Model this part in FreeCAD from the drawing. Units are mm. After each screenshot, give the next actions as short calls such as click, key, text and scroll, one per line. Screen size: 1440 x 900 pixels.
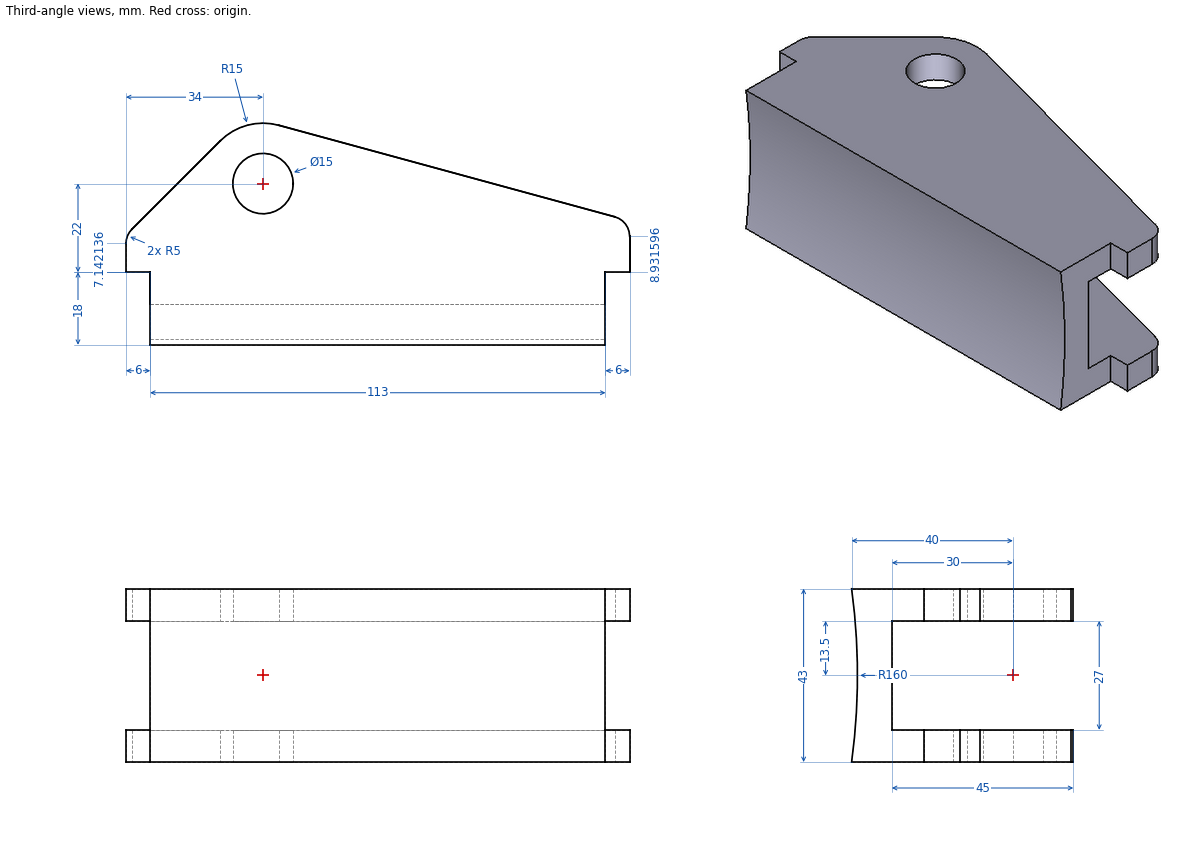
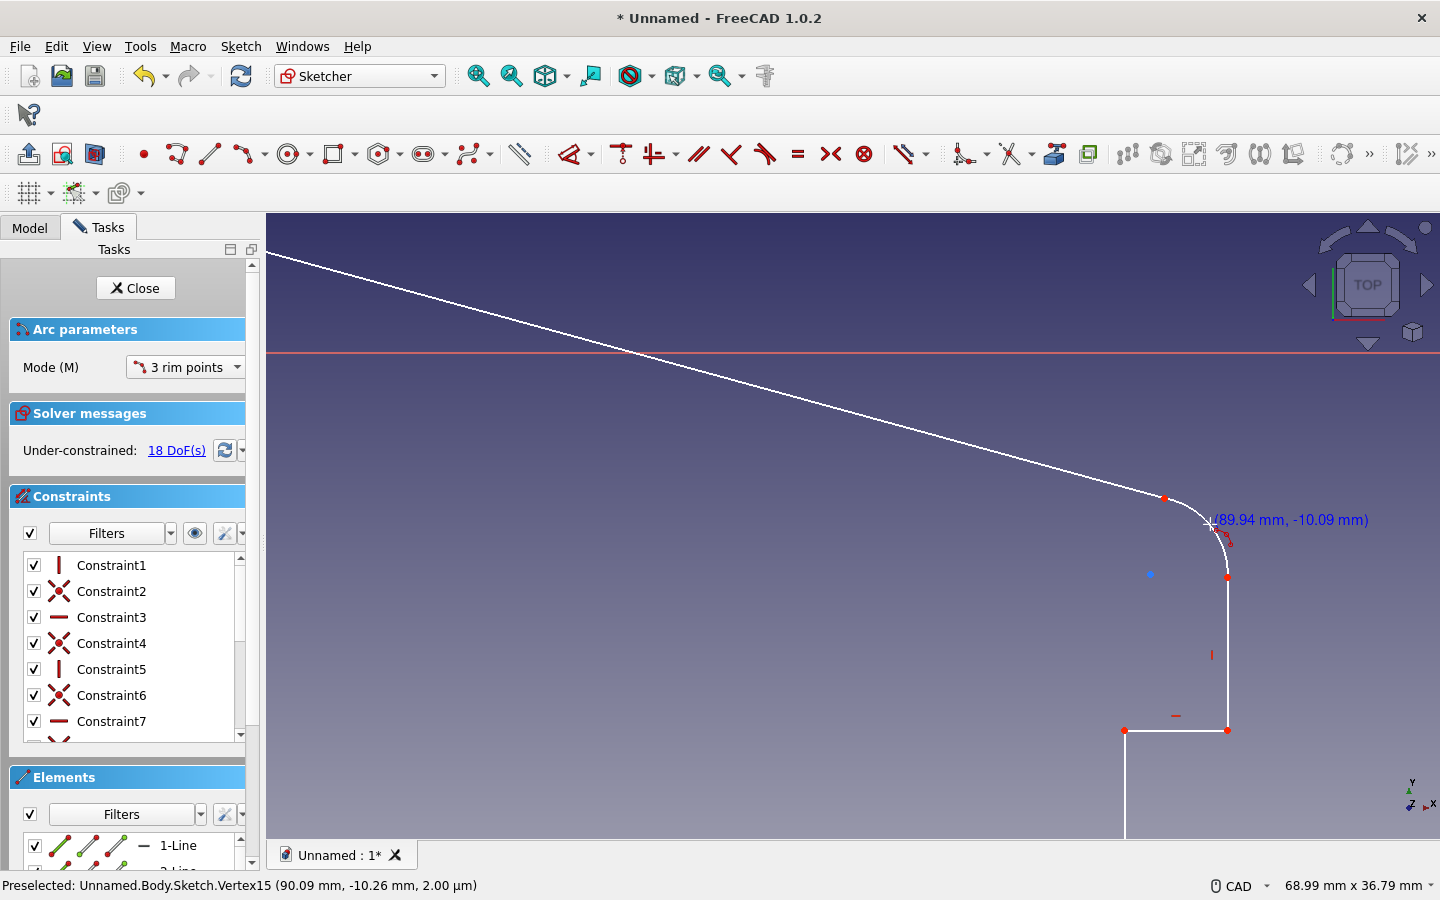
scroll(1052, 507, down, 6)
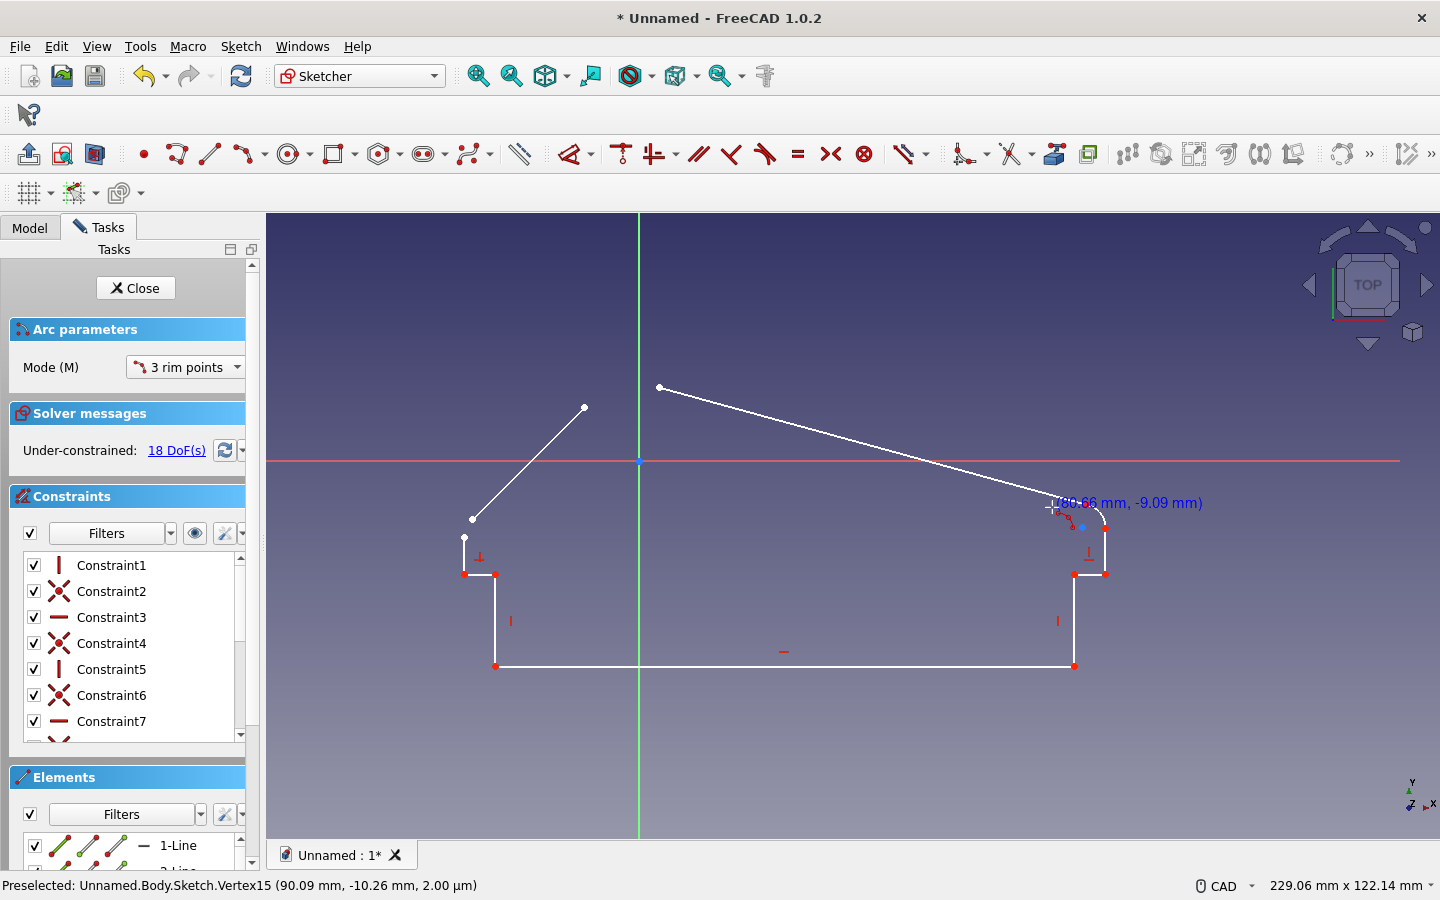
click(659, 388)
click(584, 408)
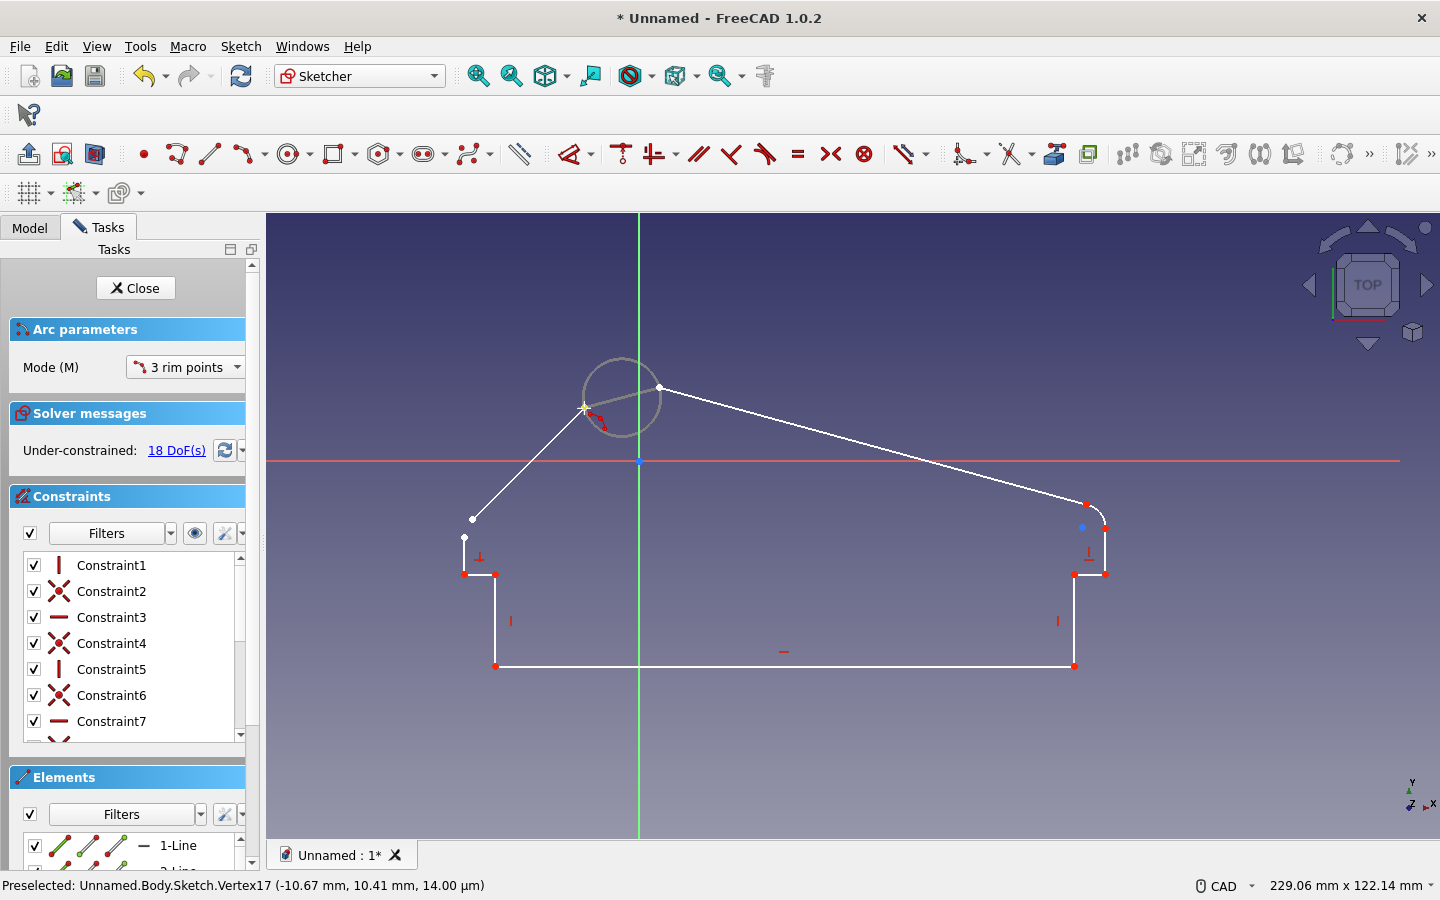
scroll(619, 387, up, 3)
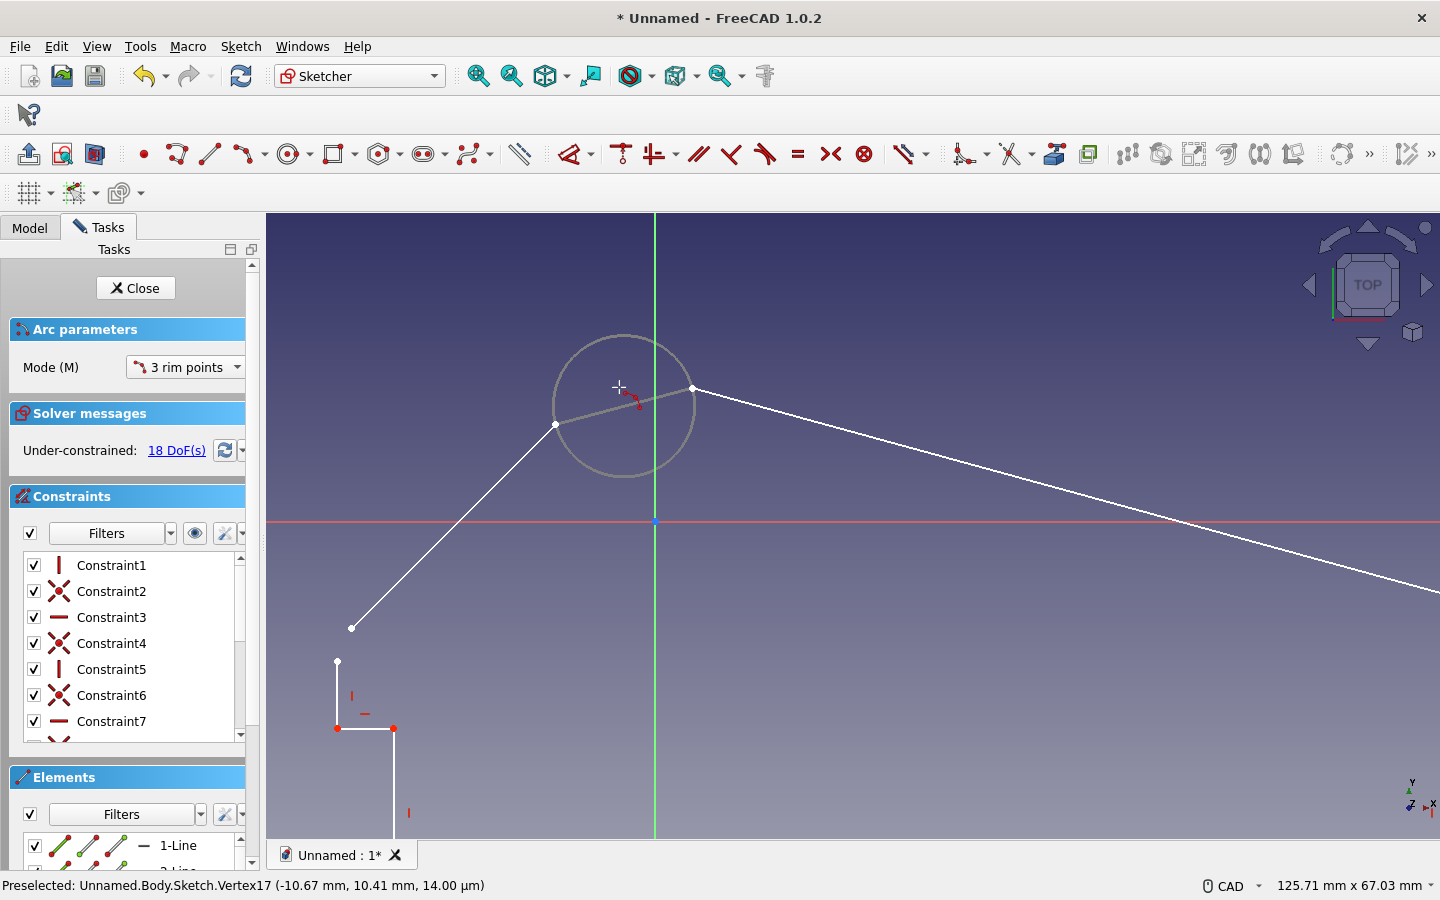
click(619, 386)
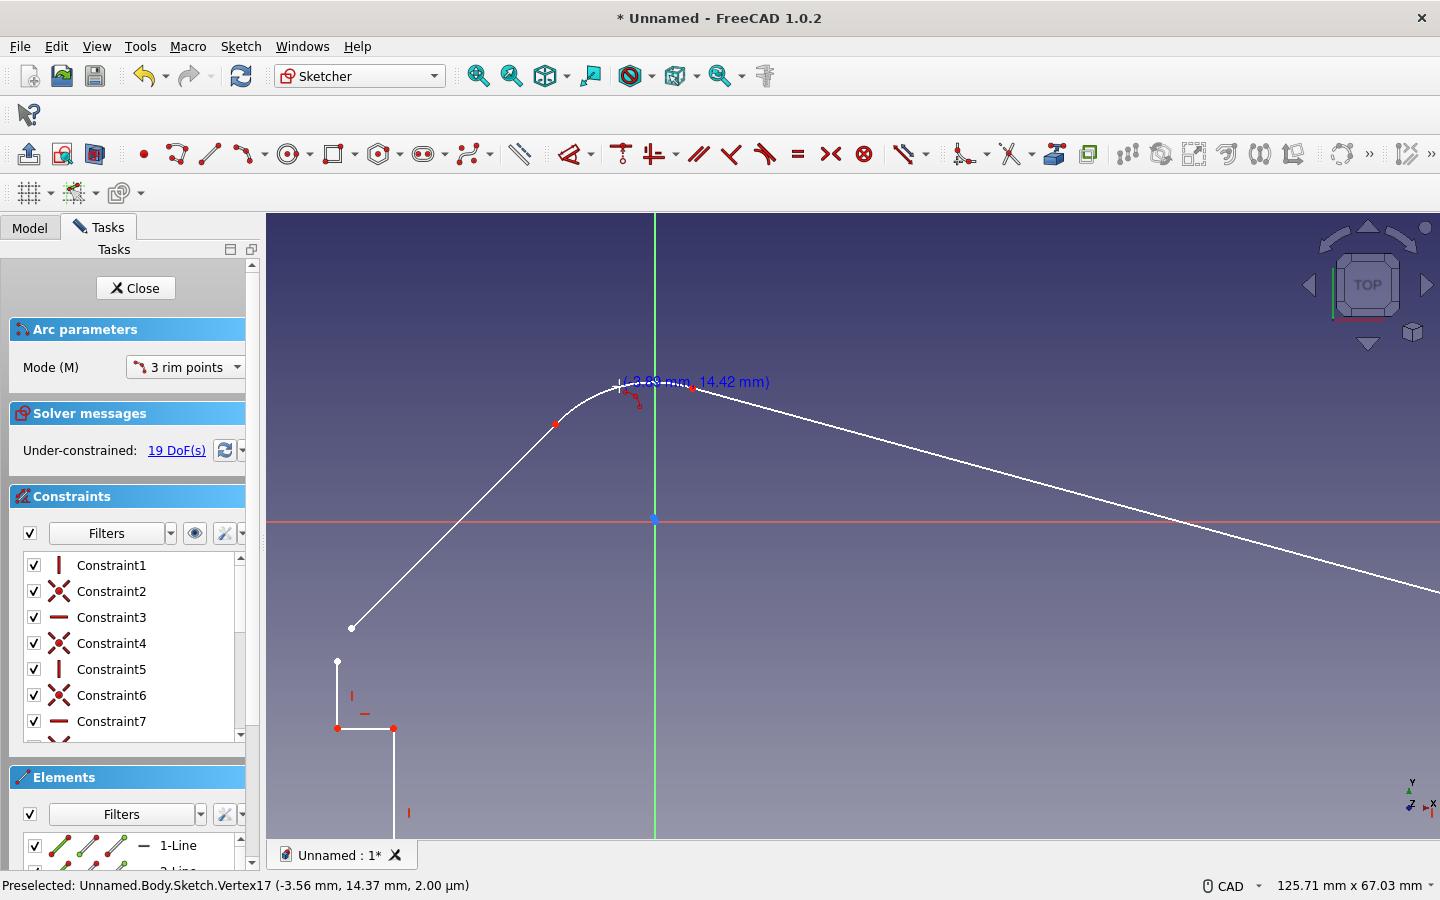
click(352, 629)
click(337, 661)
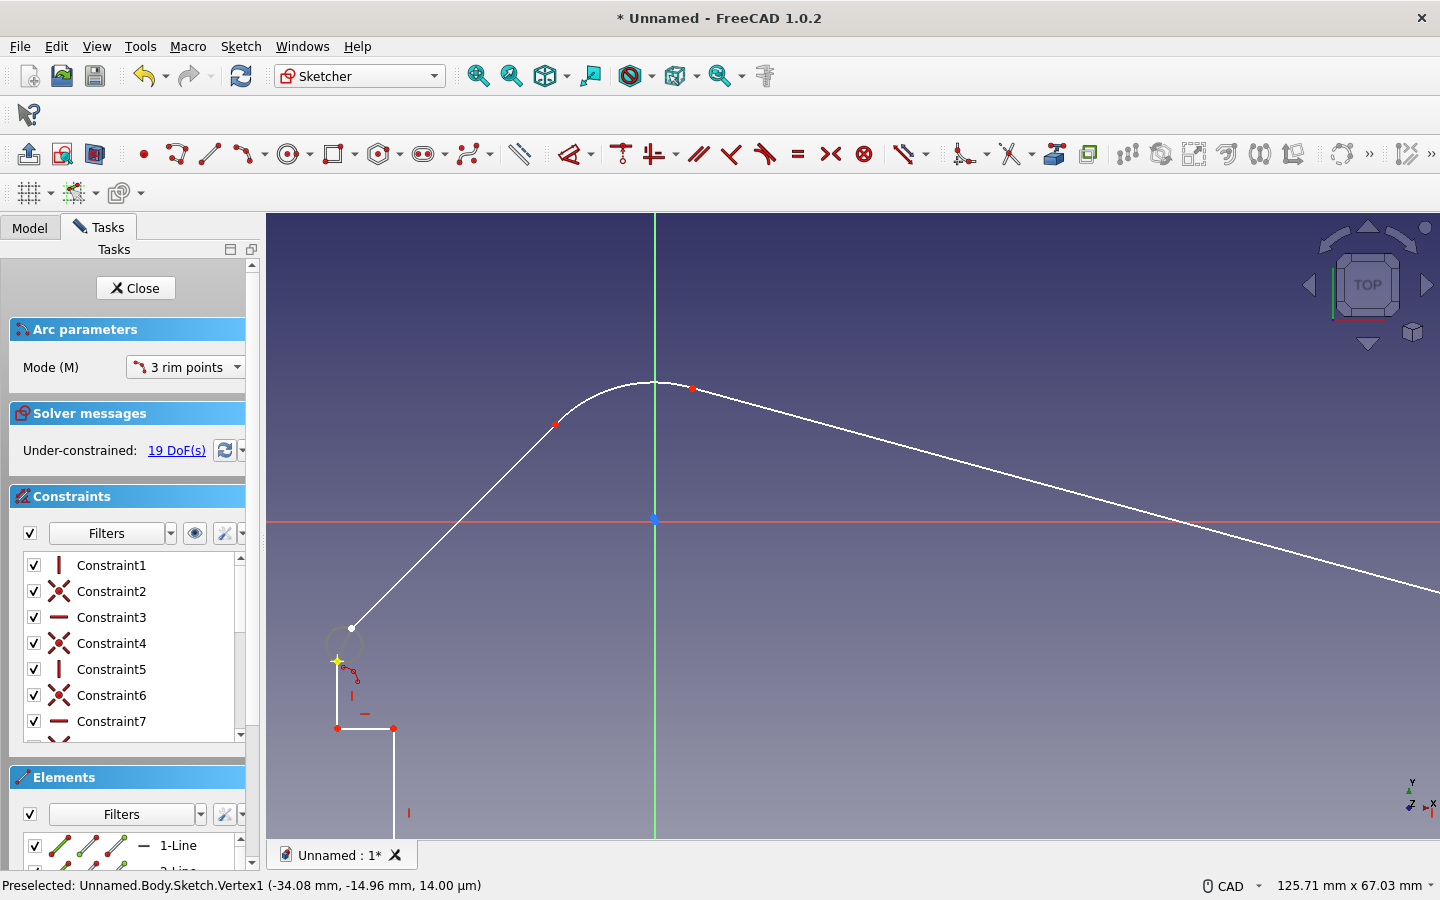
scroll(341, 643, up, 8)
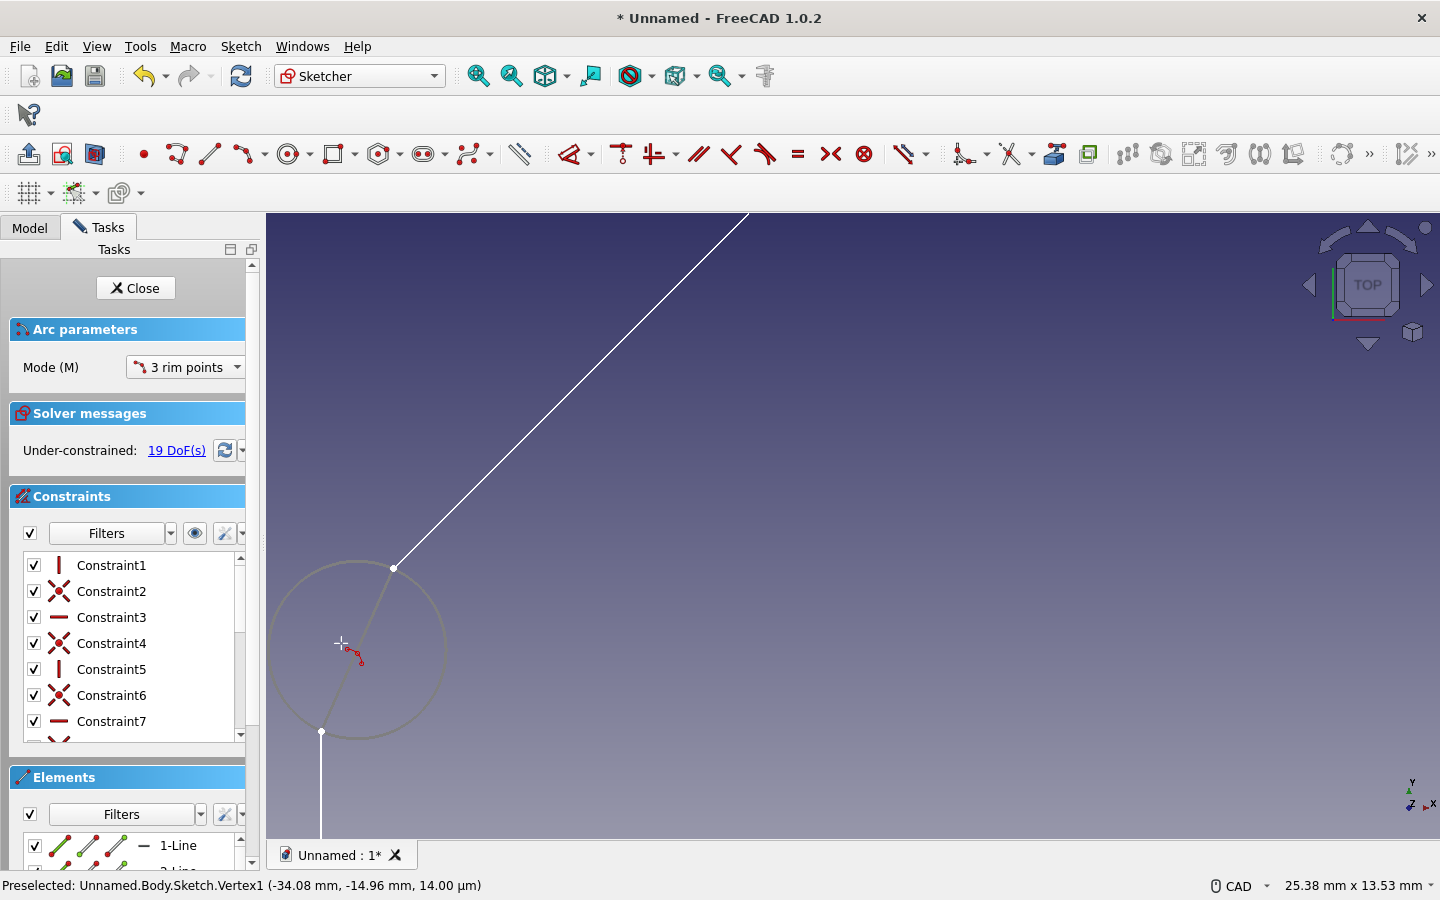
click(343, 638)